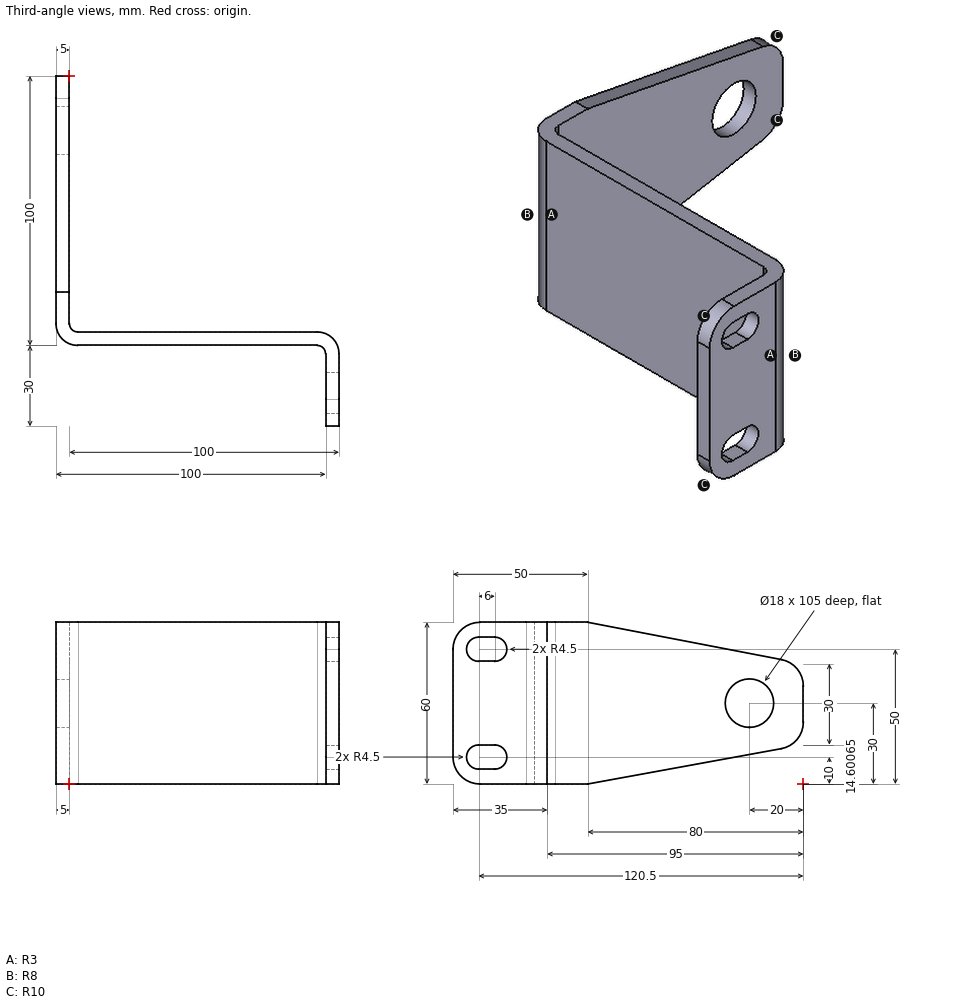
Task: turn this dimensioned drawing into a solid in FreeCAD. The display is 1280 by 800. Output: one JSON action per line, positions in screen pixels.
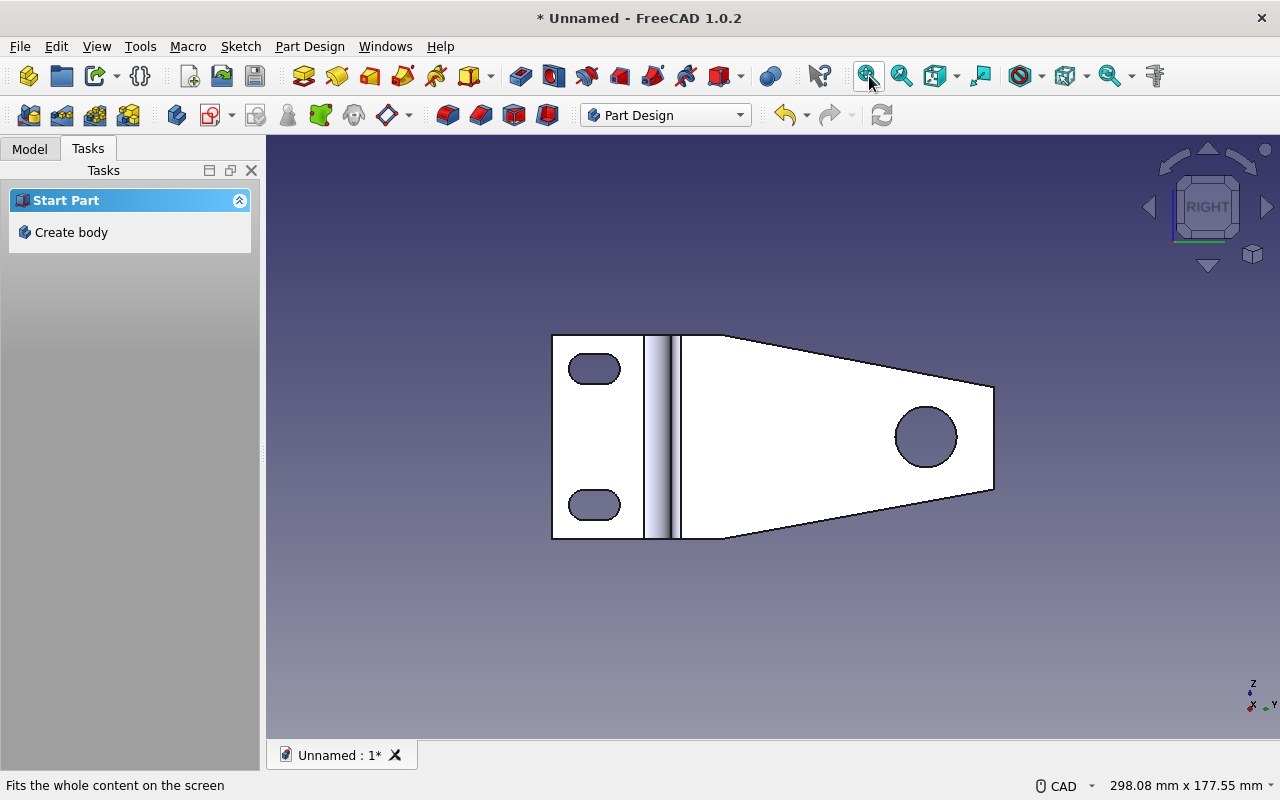
{"action": "scroll", "coordinate": [994, 386], "scroll_direction": "up", "scroll_amount": 5}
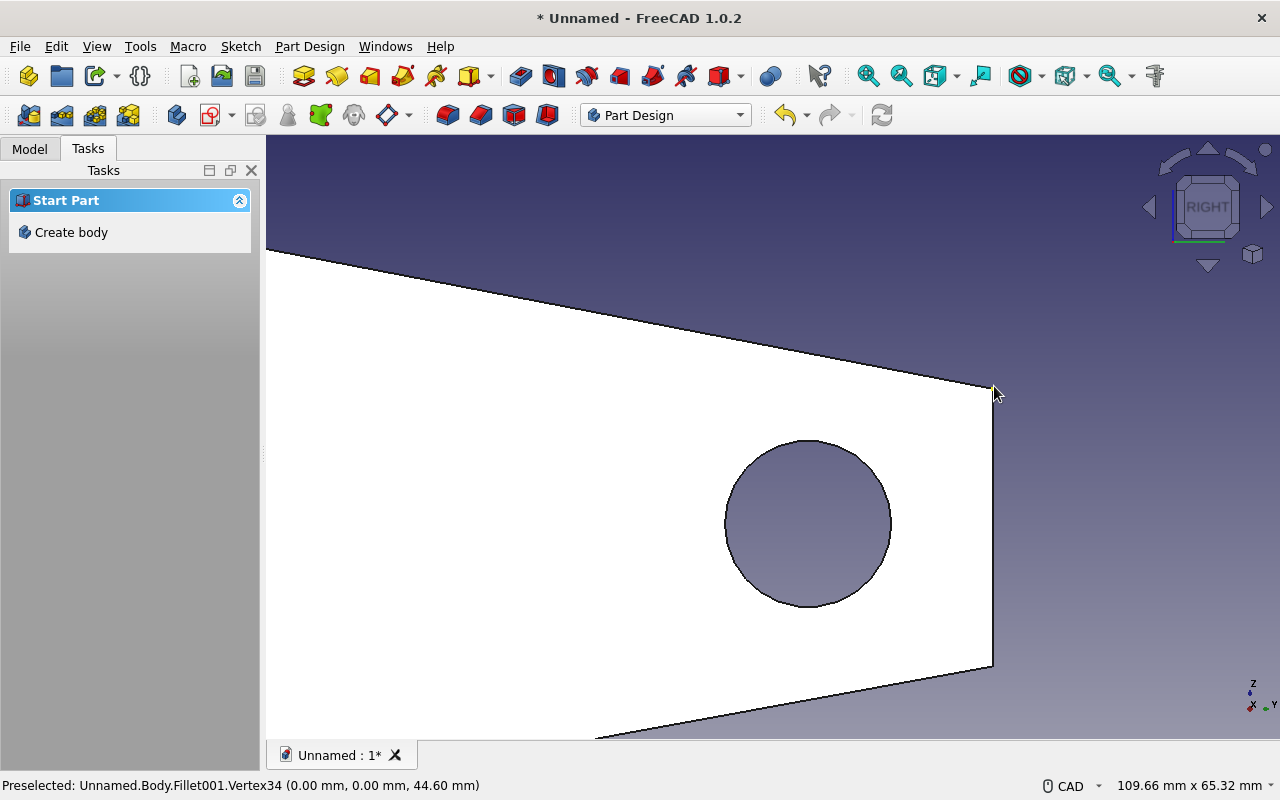
{"action": "left_click", "coordinate": [869, 76]}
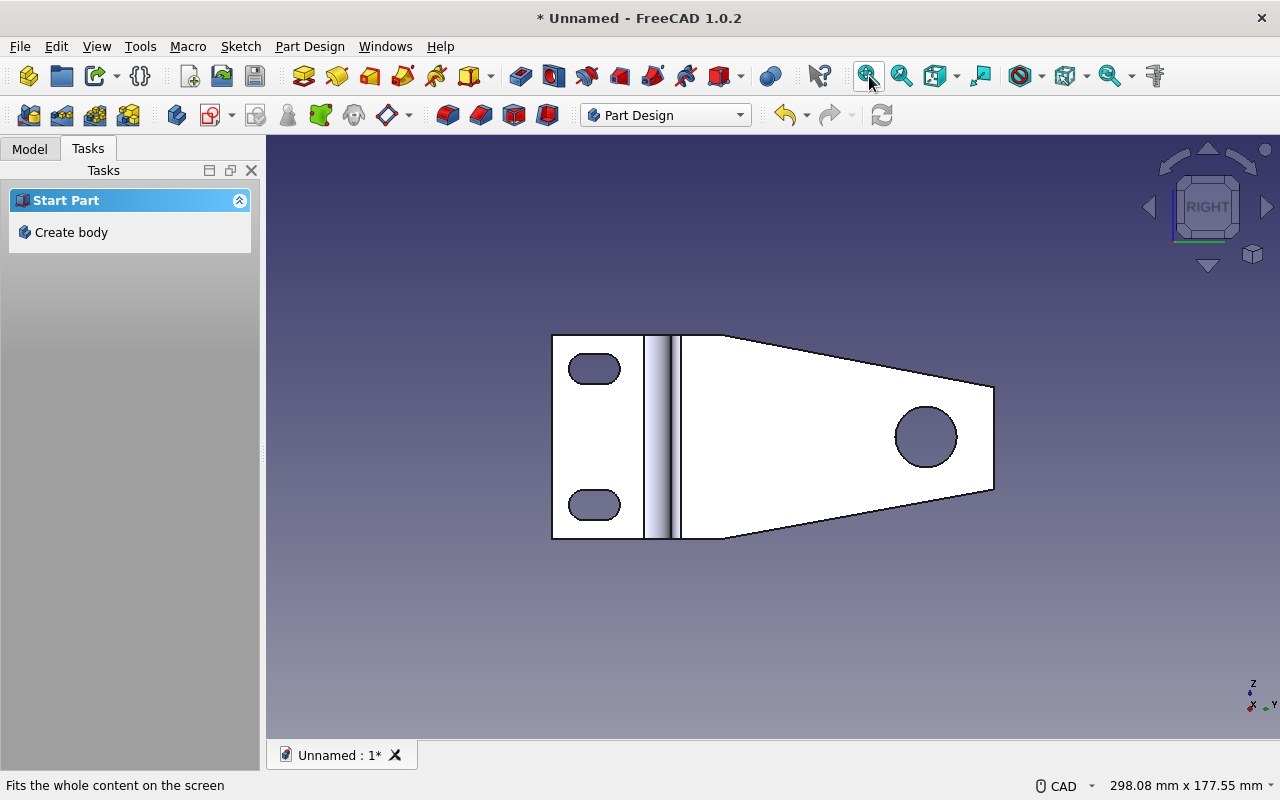
{"action": "key", "text": "0"}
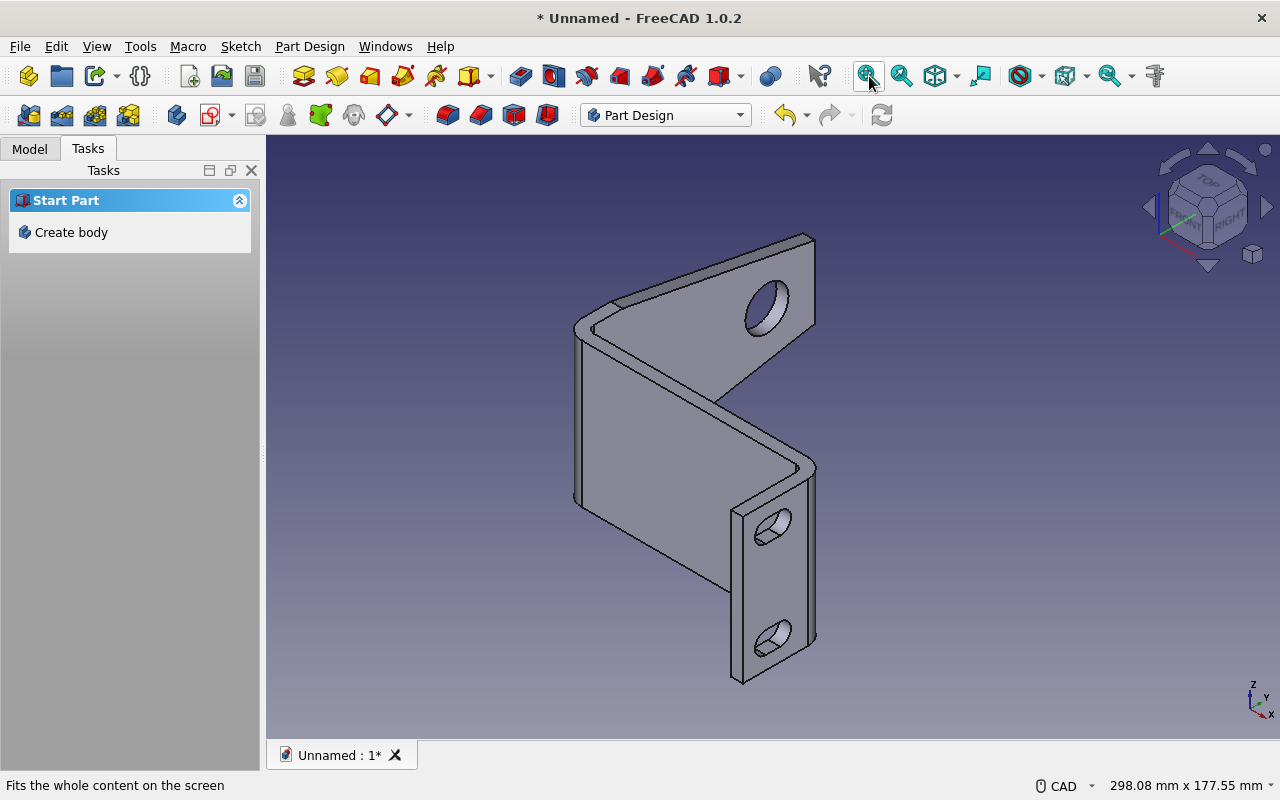
{"action": "left_click", "coordinate": [737, 512]}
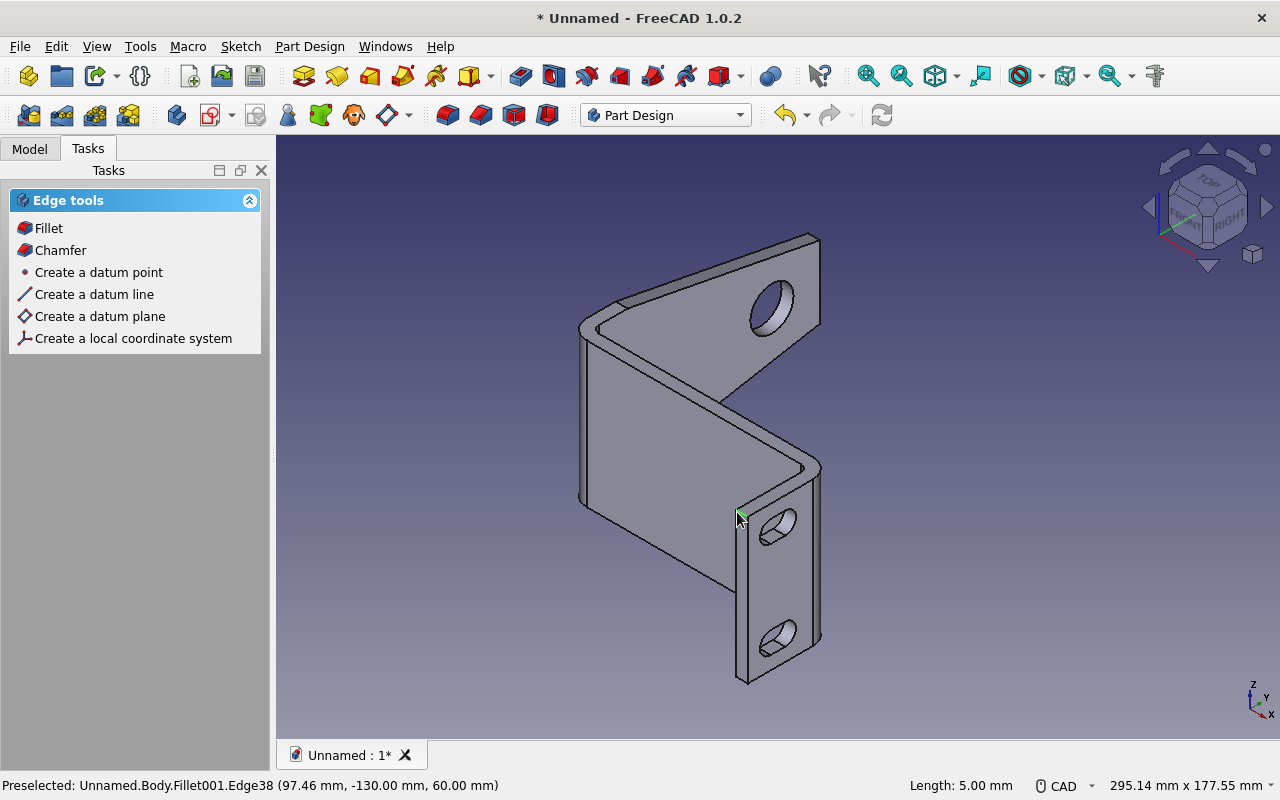
{"action": "scroll", "coordinate": [814, 236], "scroll_direction": "up", "scroll_amount": 5}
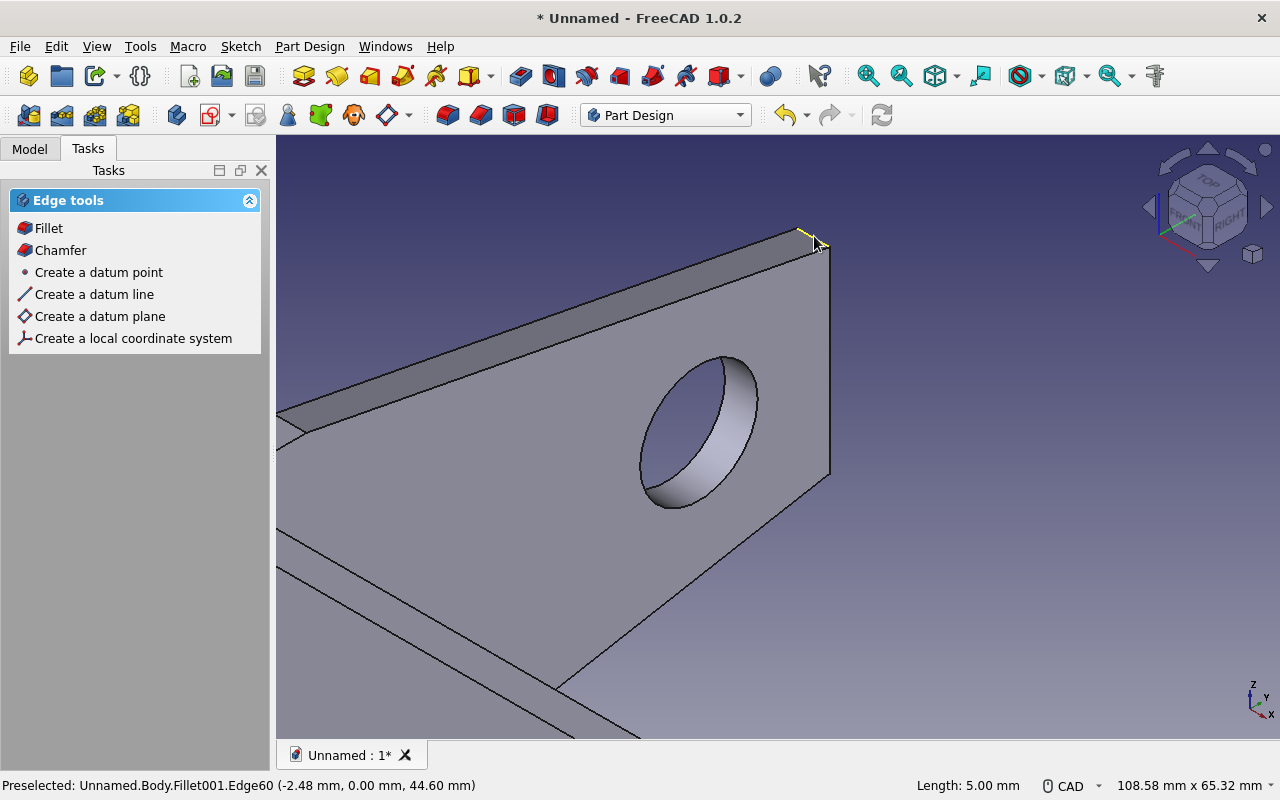
{"action": "left_click", "coordinate": [869, 76]}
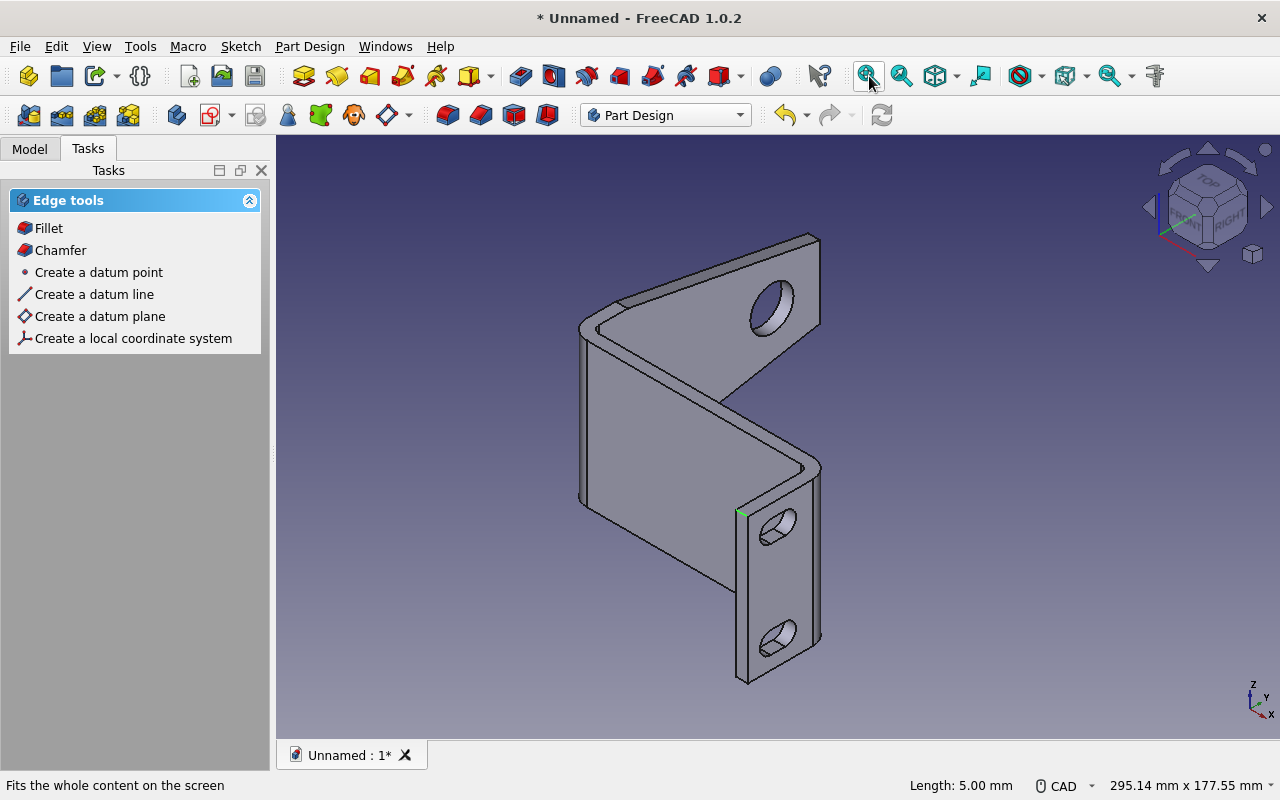
{"action": "key", "text": "2"}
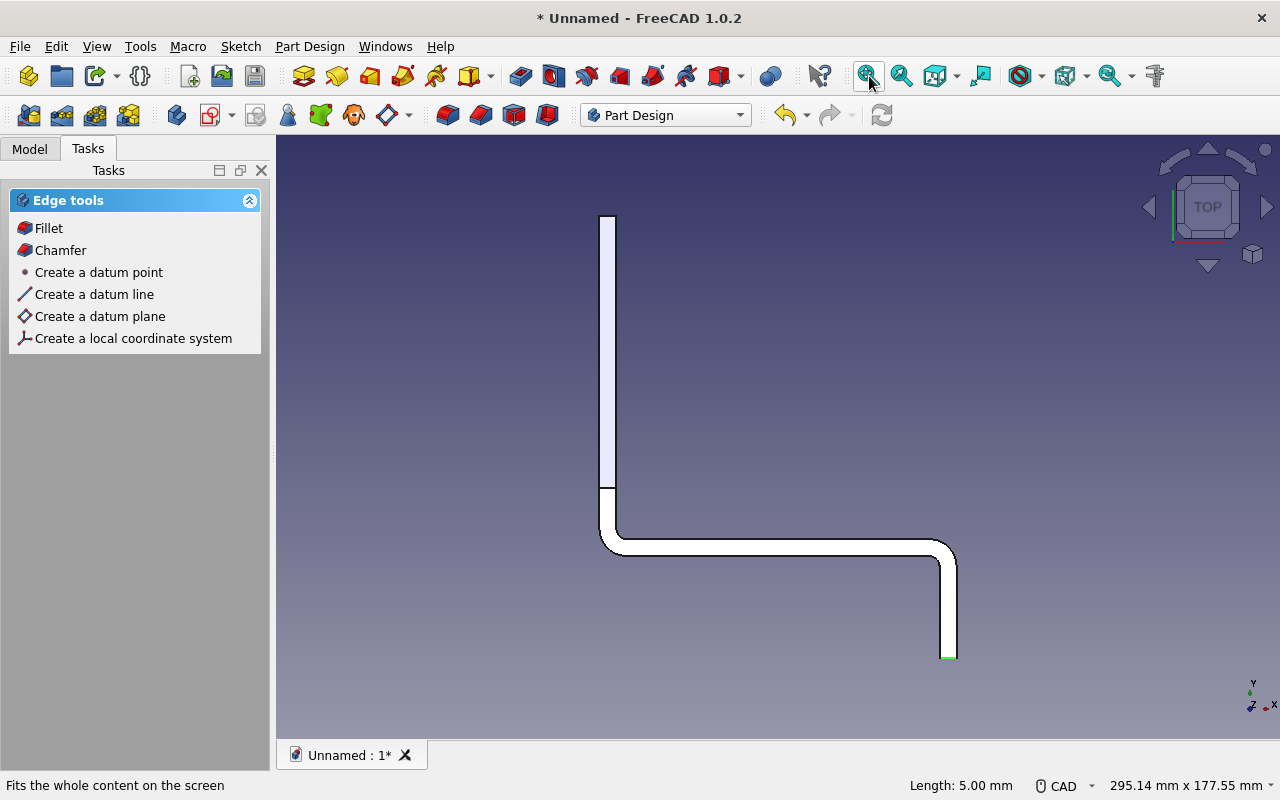
{"action": "scroll", "coordinate": [608, 215], "scroll_direction": "up", "scroll_amount": 5}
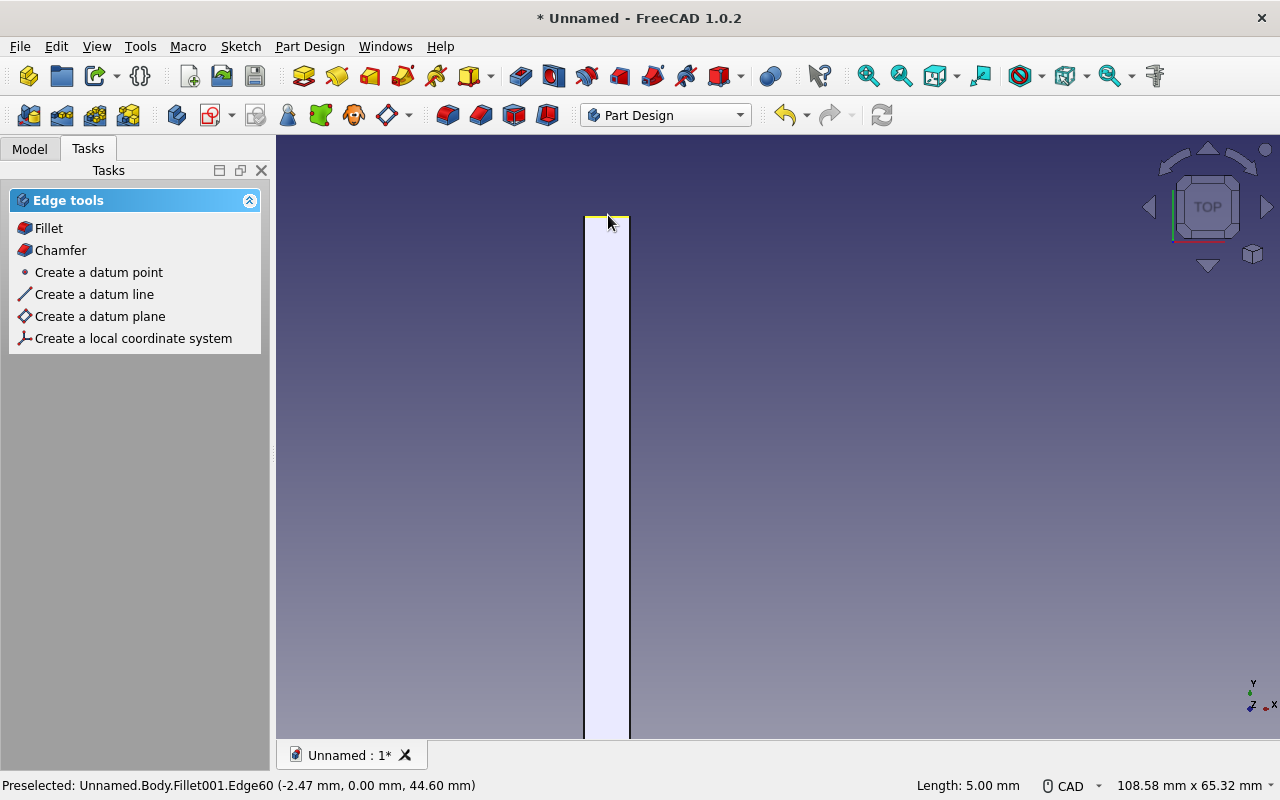
{"action": "left_click", "coordinate": [869, 76]}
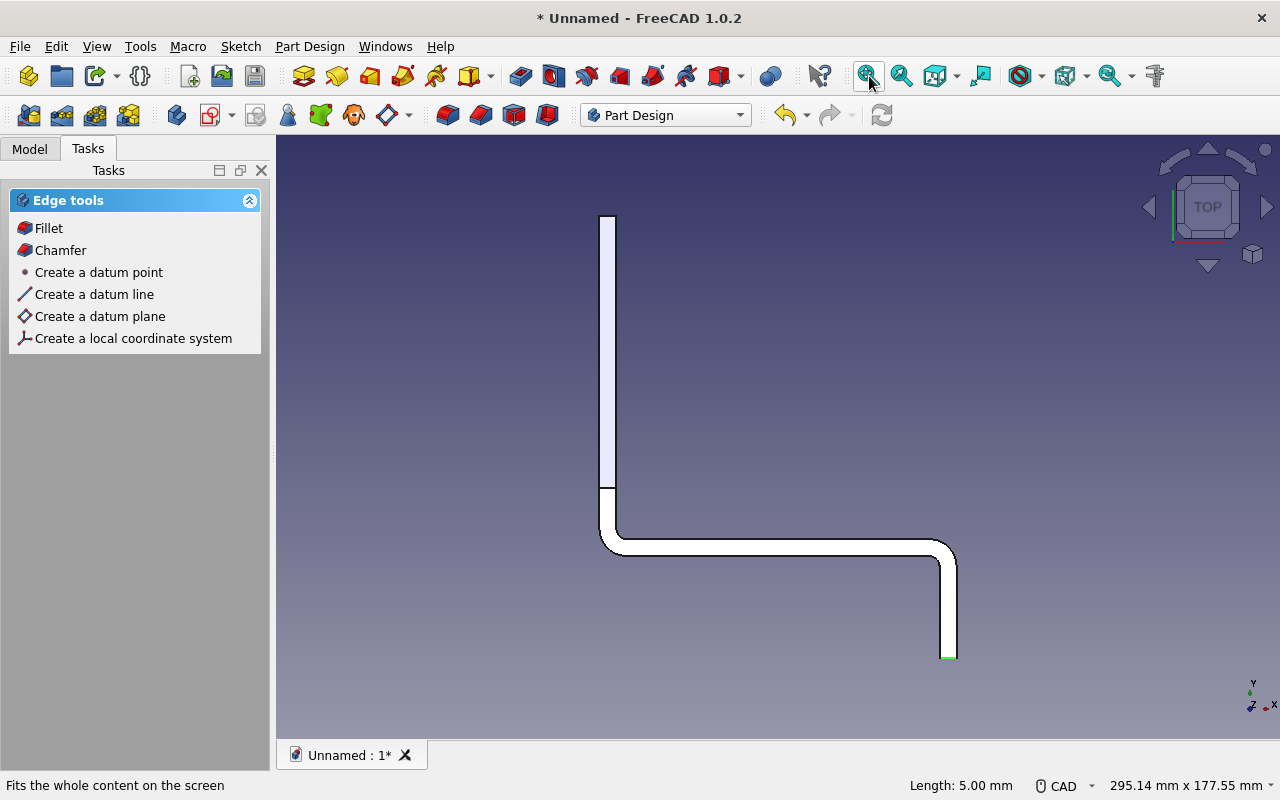
{"action": "key", "text": "1"}